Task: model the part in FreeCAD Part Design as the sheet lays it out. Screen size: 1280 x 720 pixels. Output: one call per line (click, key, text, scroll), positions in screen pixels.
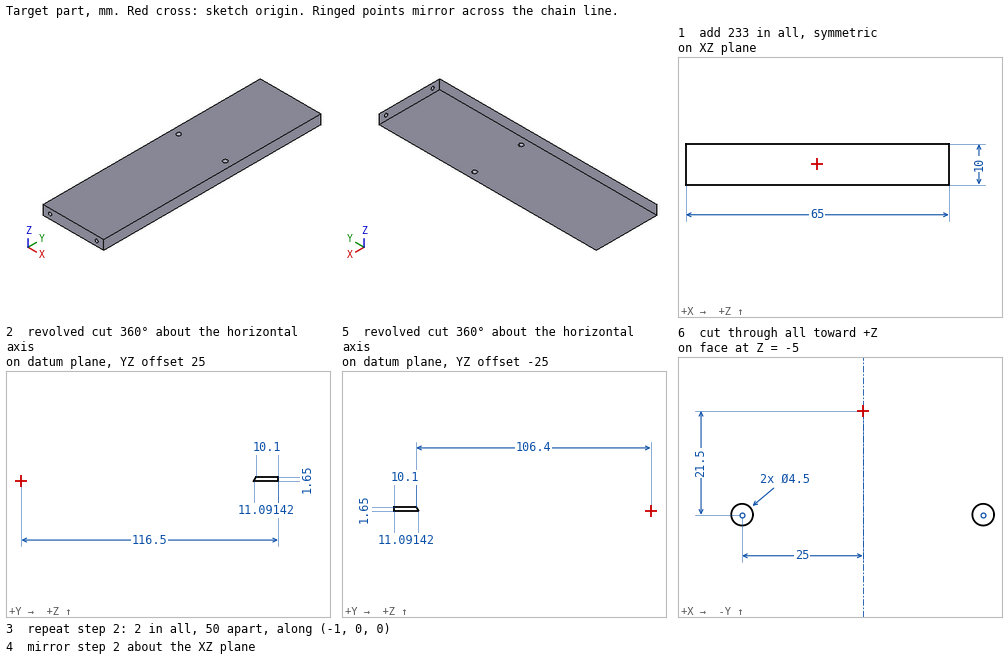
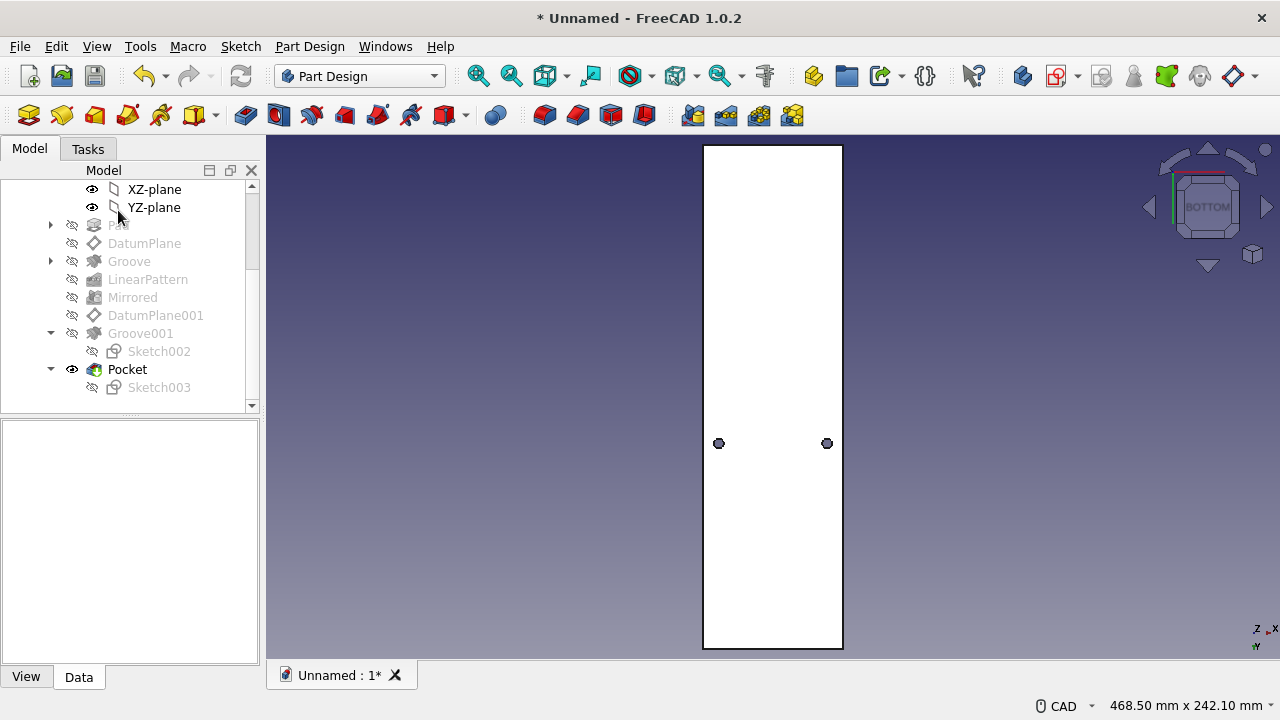
key(0)